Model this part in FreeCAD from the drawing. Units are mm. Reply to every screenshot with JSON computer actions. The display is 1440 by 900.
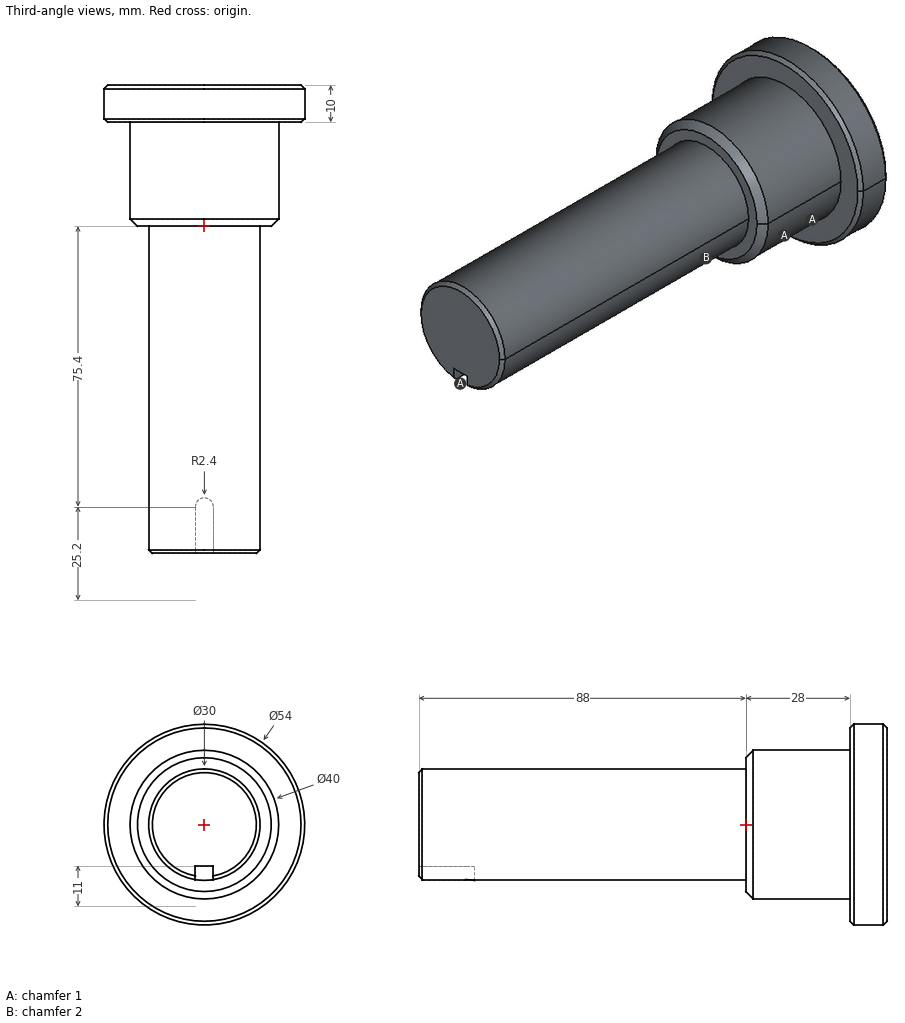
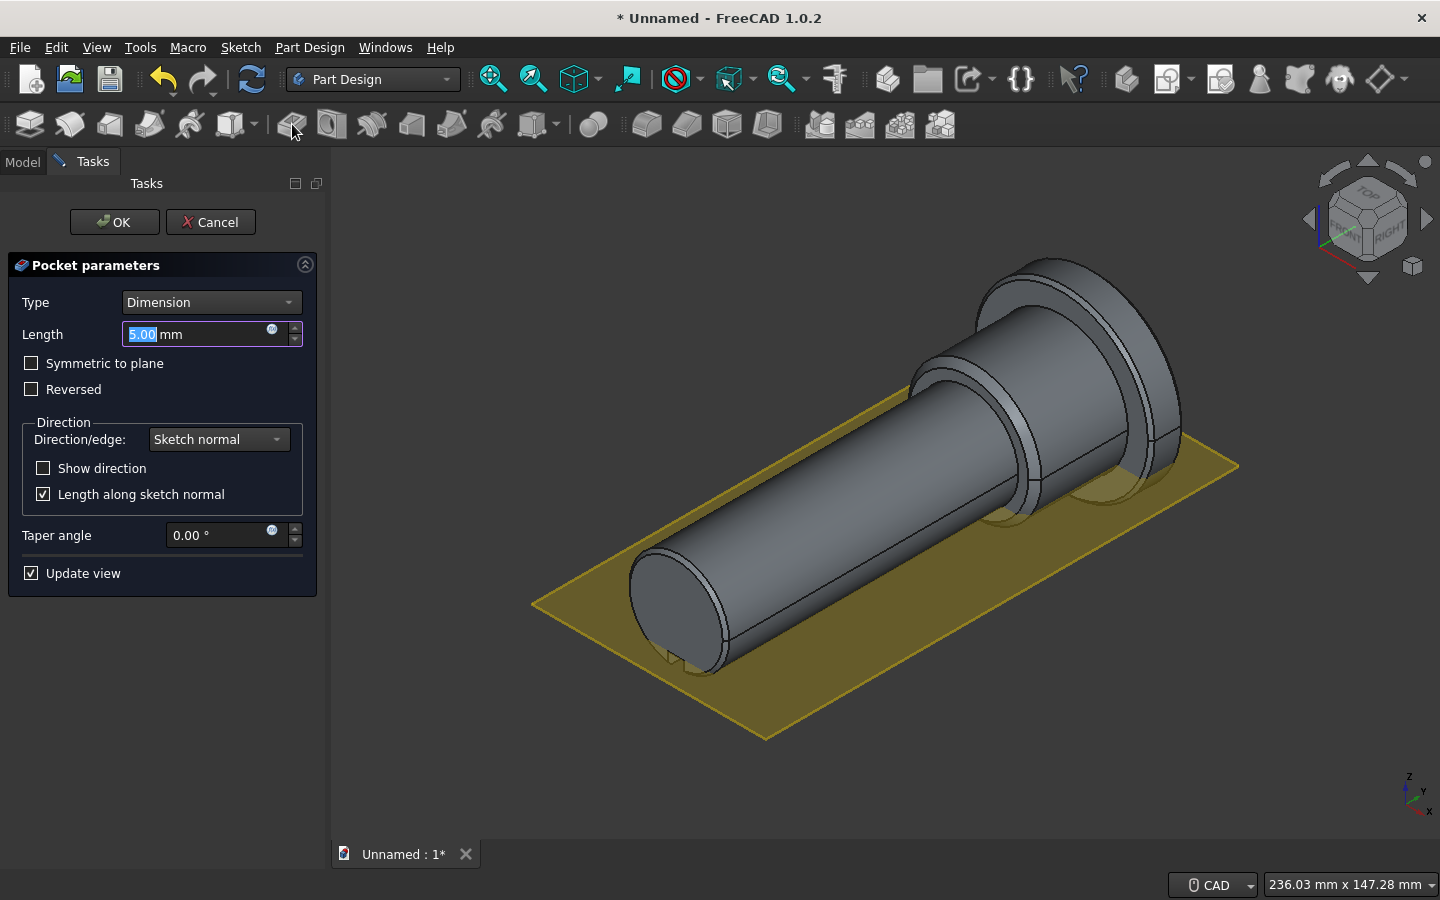
{"action": "type", "text": "11"}
{"action": "key", "text": "Tab"}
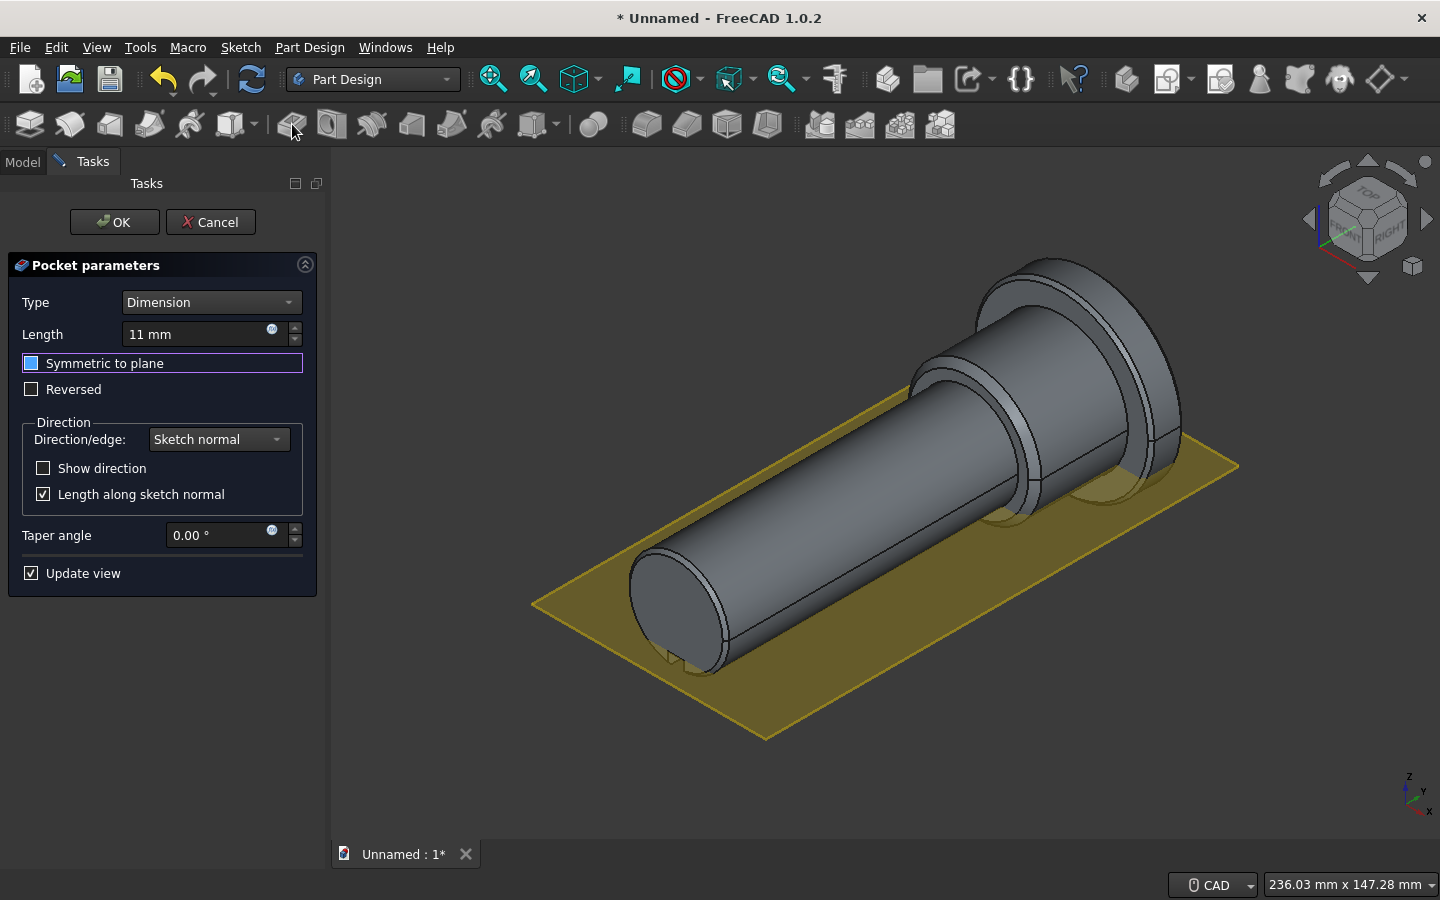
{"action": "left_click", "coordinate": [115, 222]}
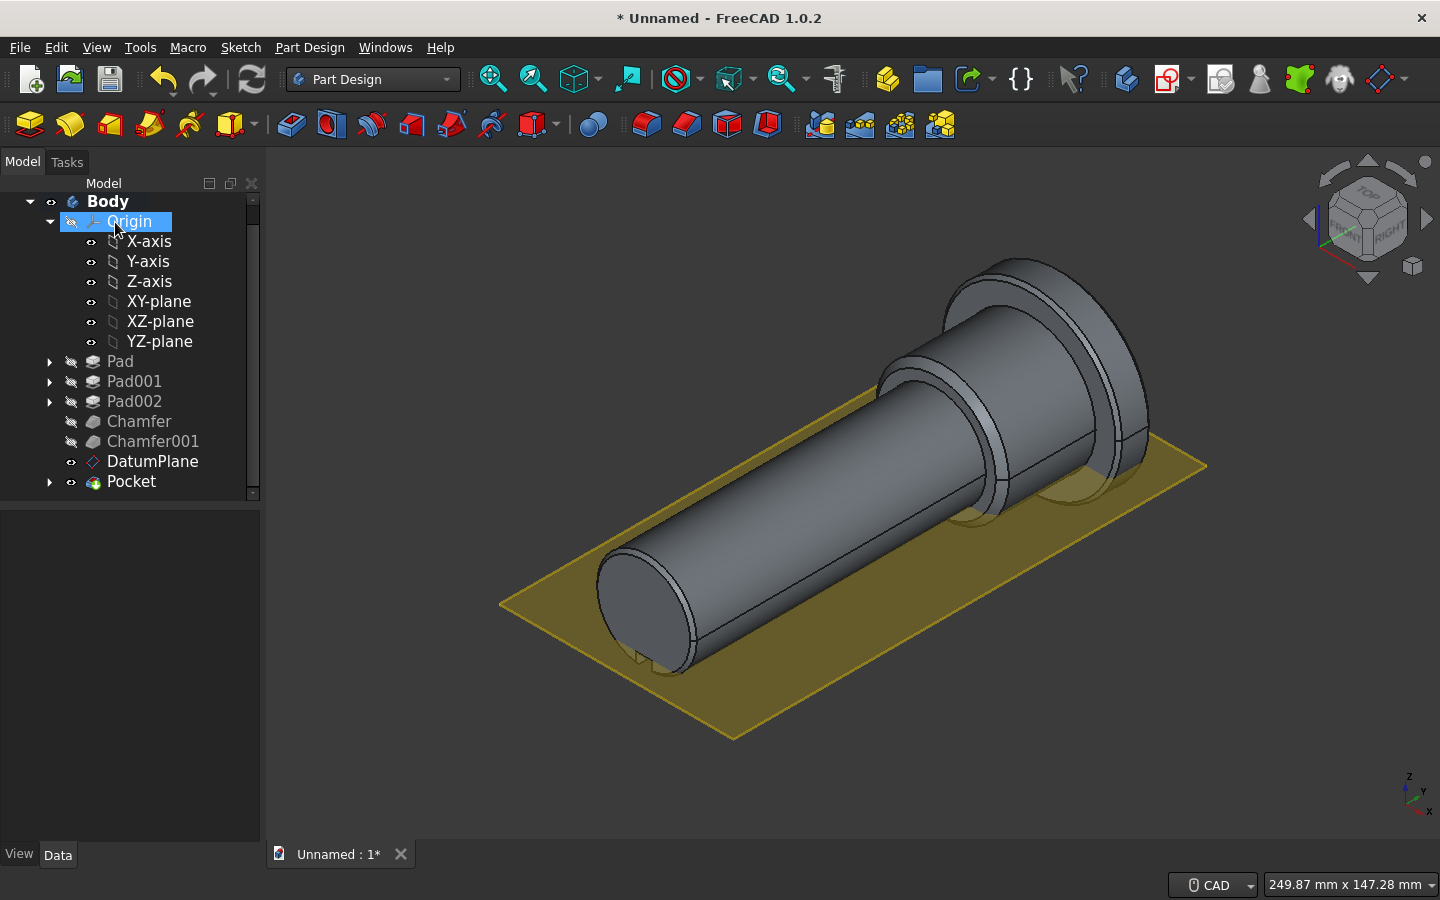
{"action": "left_click", "coordinate": [116, 462]}
{"action": "key", "text": "space"}